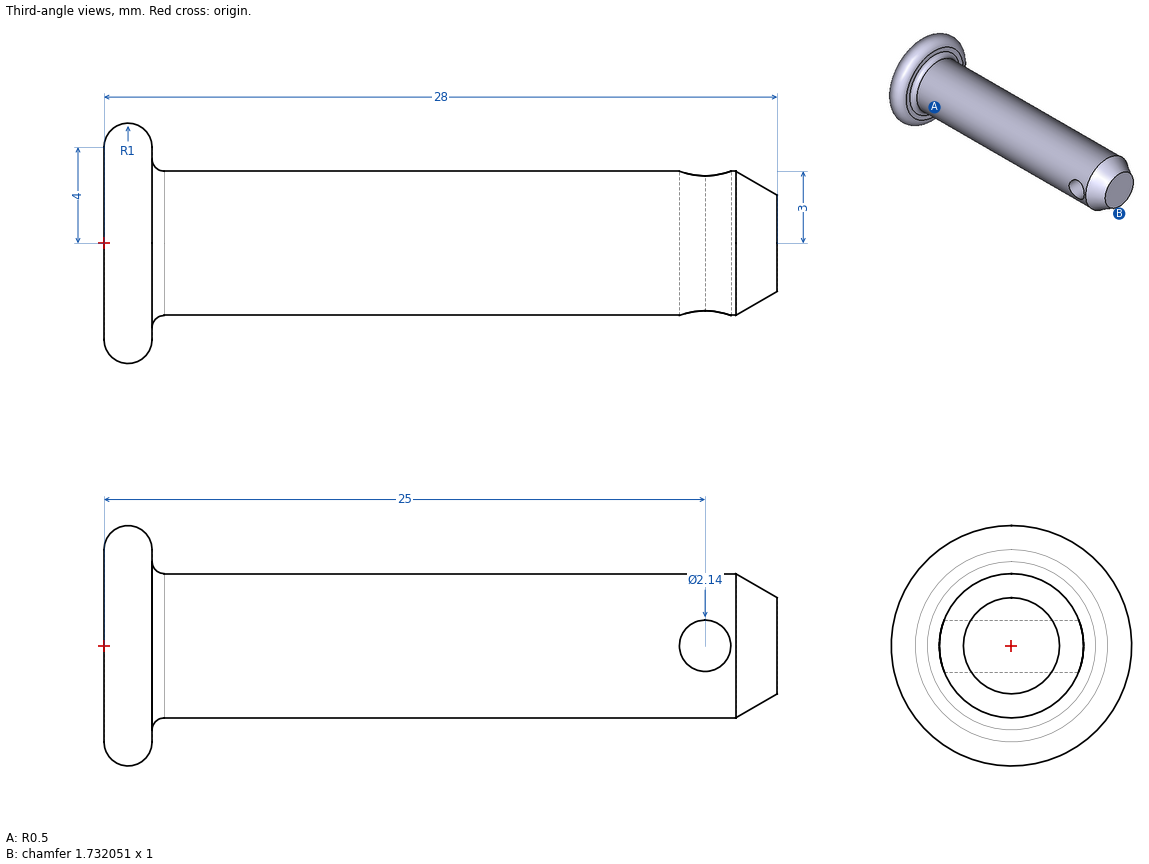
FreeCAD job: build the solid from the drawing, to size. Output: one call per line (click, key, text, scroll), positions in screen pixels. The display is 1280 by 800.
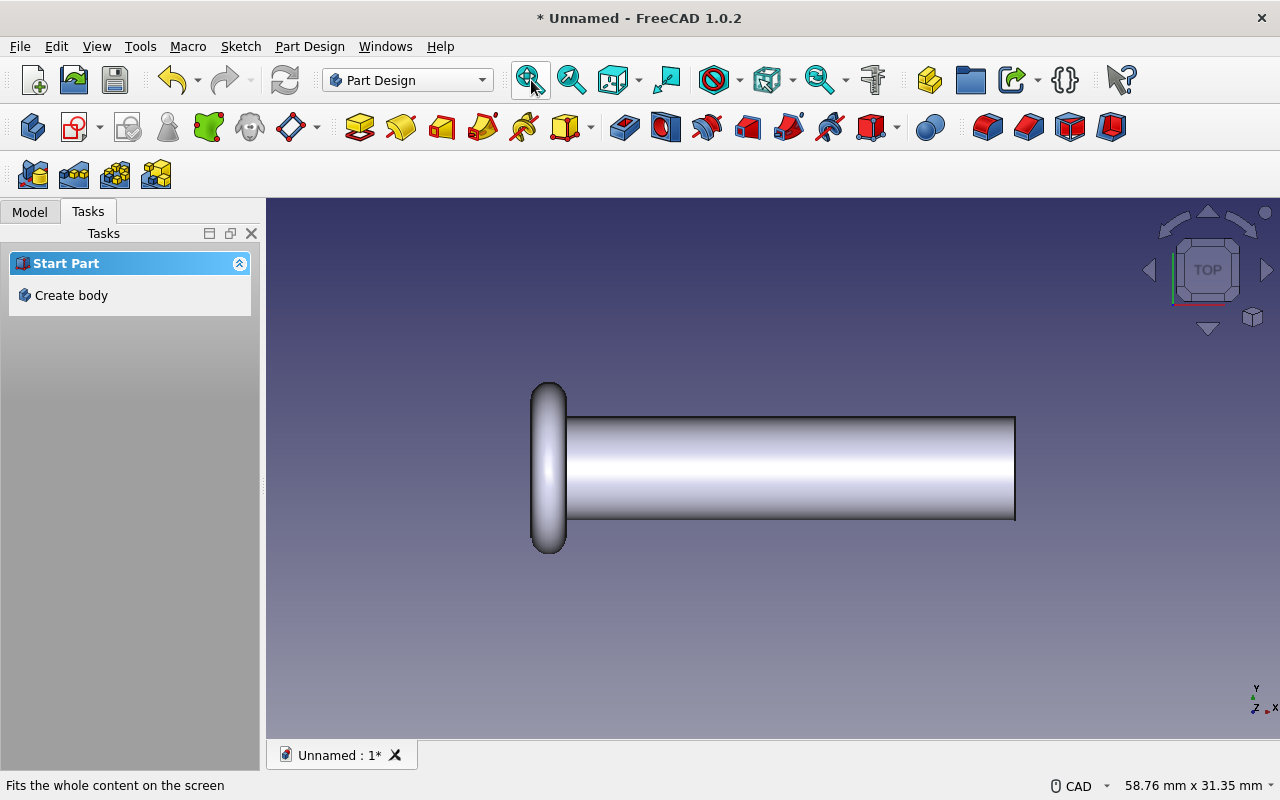
key(1)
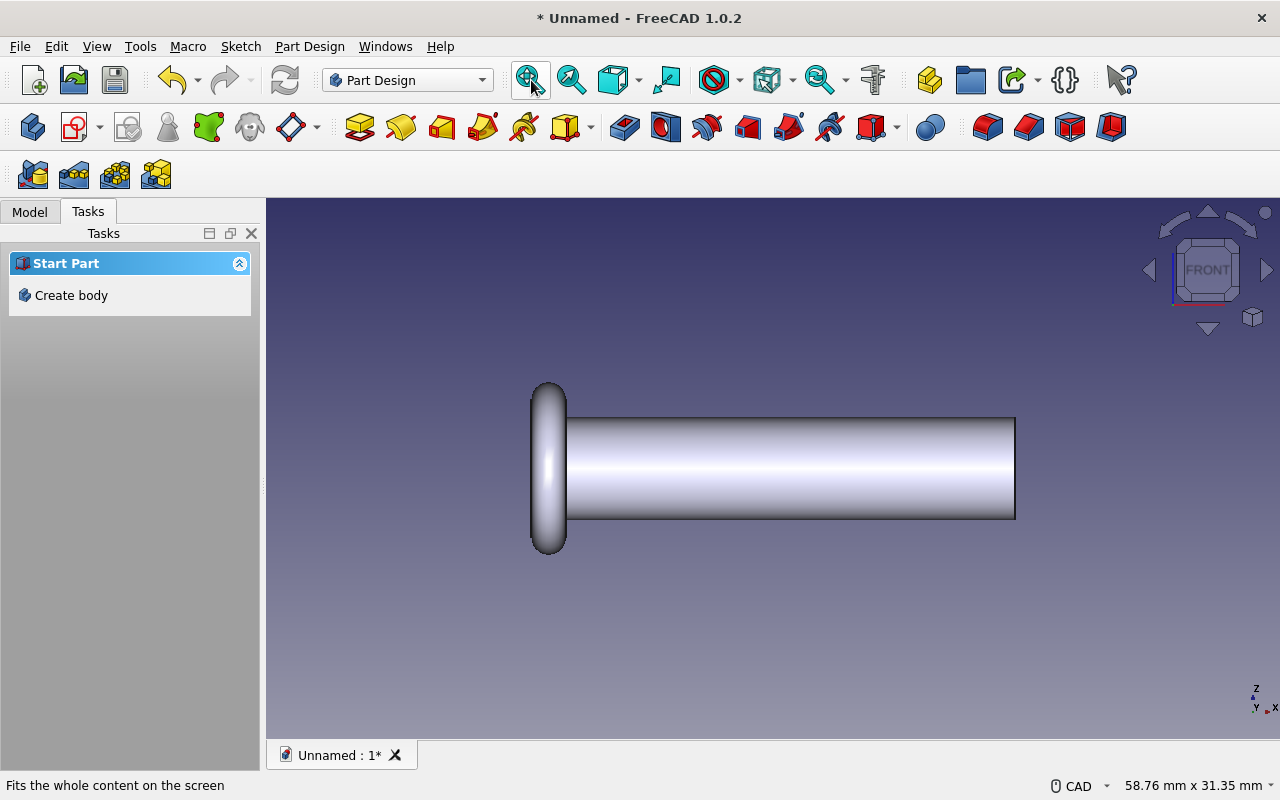
key(3)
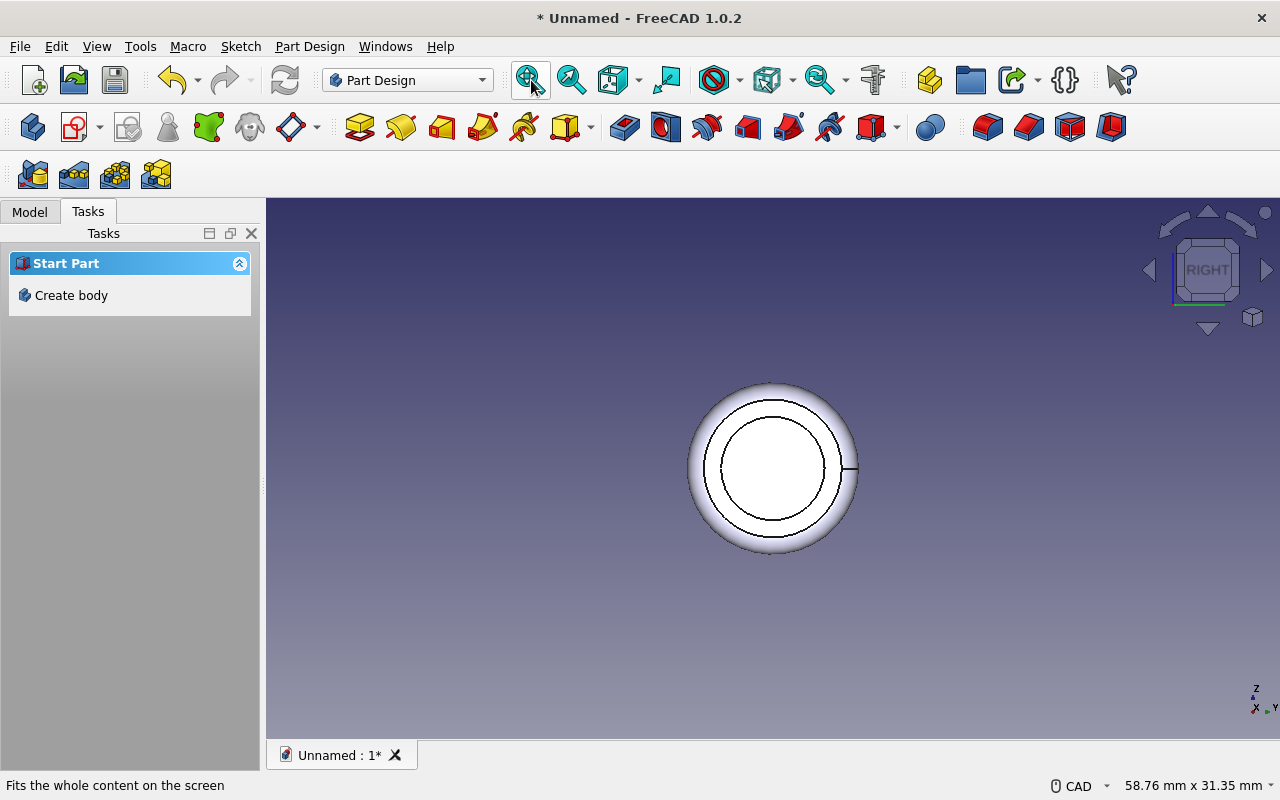
click(531, 80)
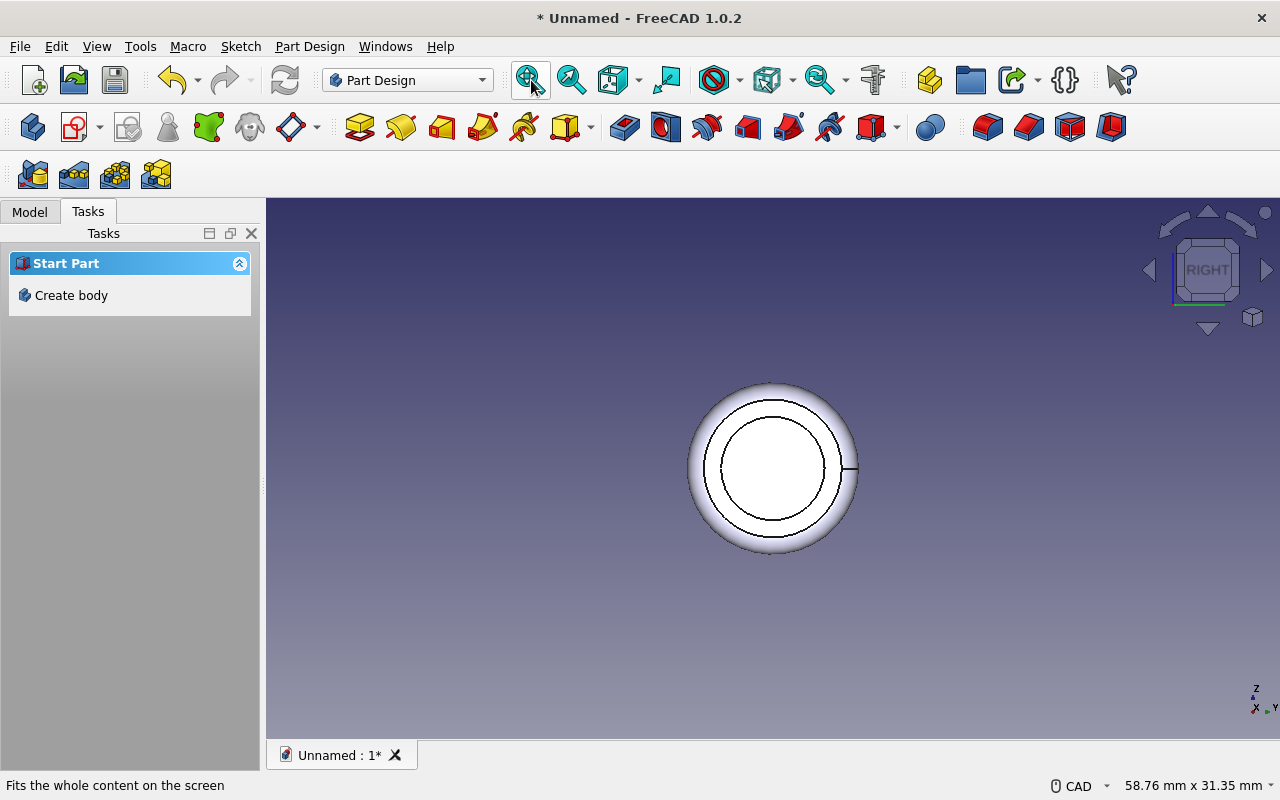
key(5)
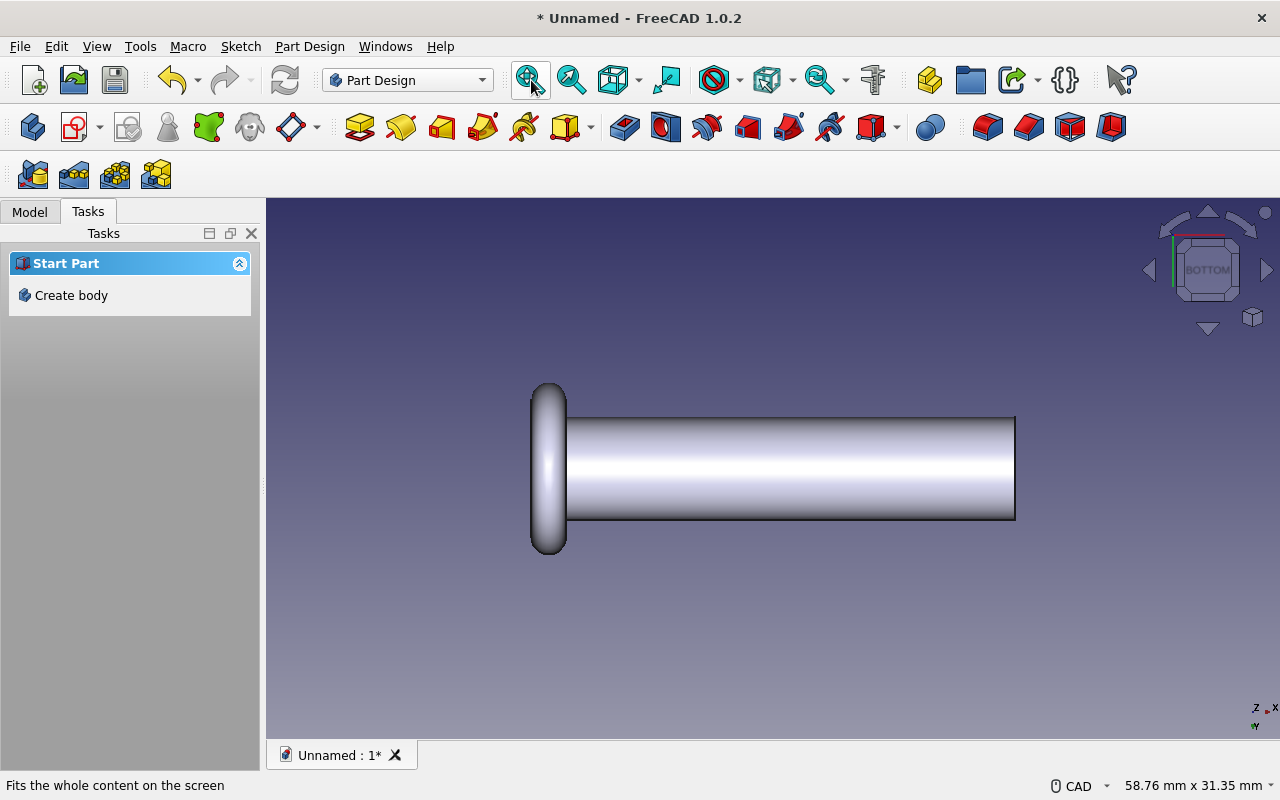
key(4)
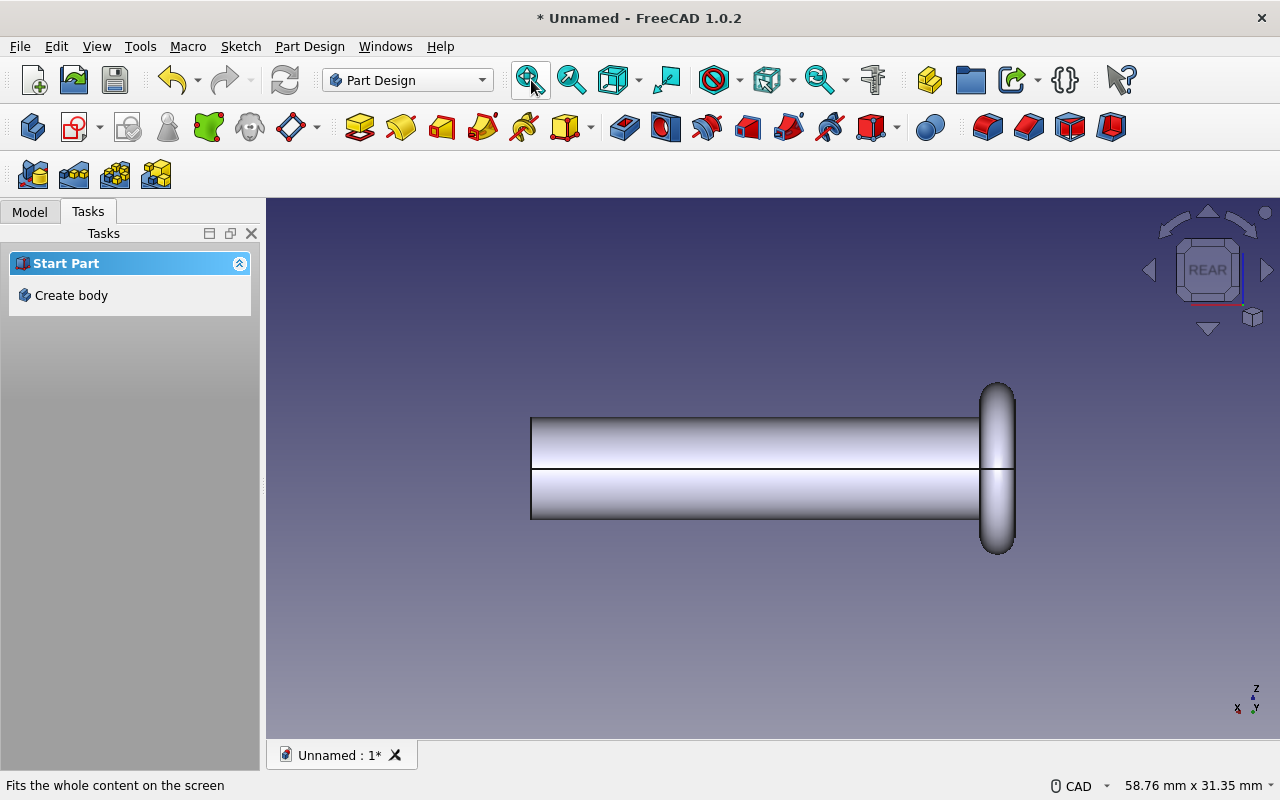
key(6)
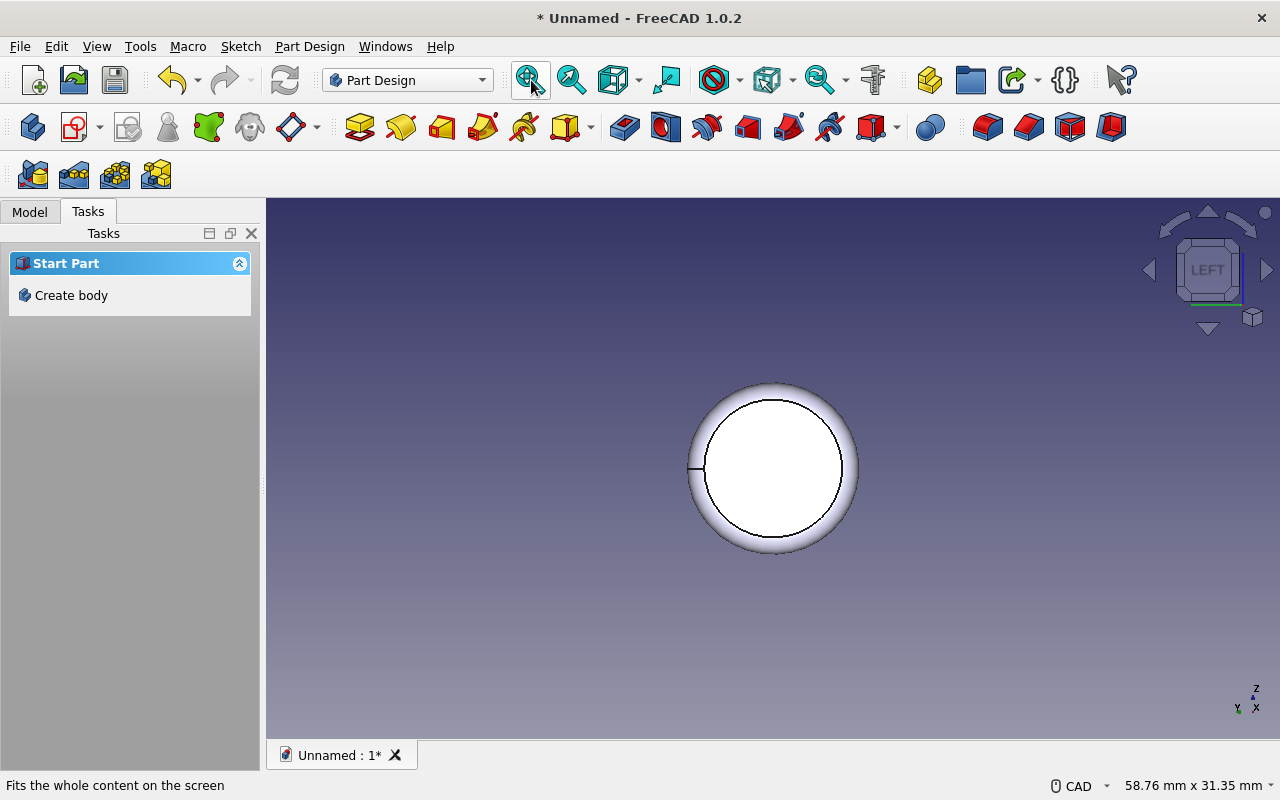
key(v)
key(f)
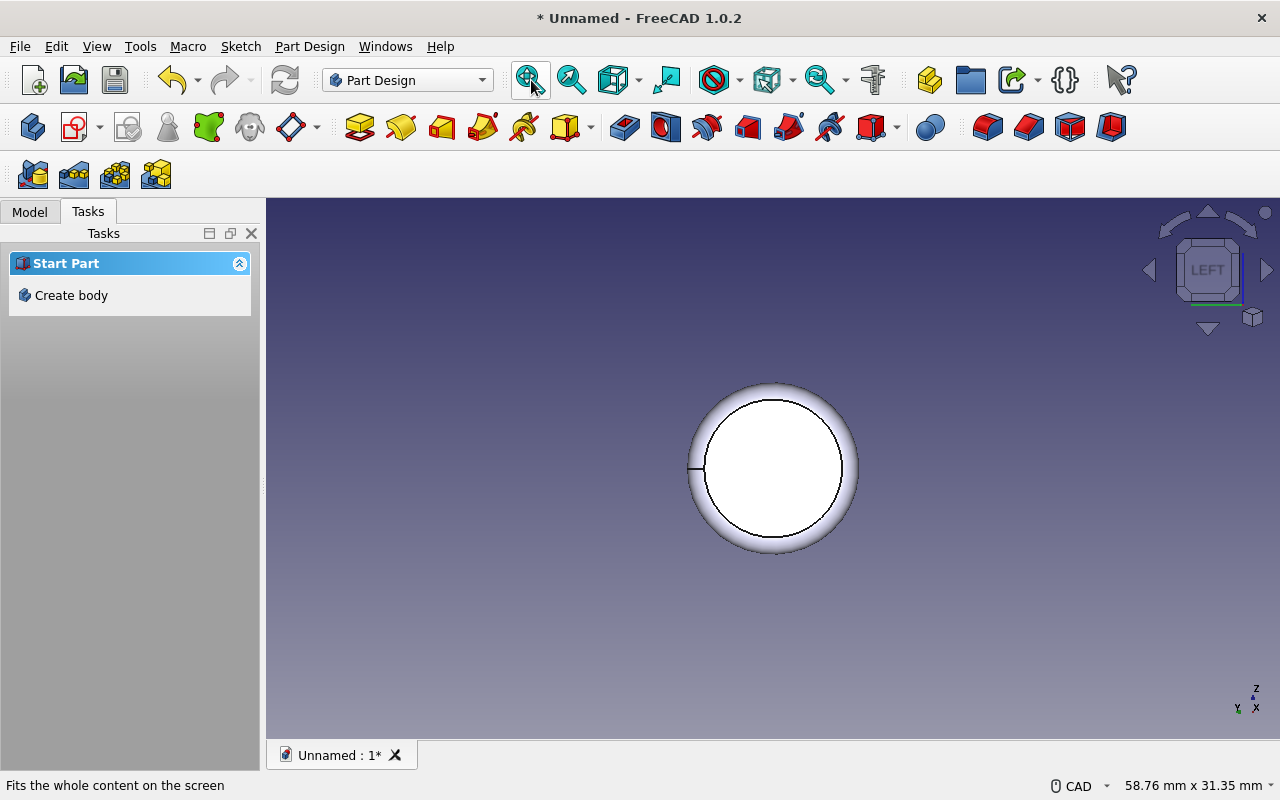
key(v)
key(3)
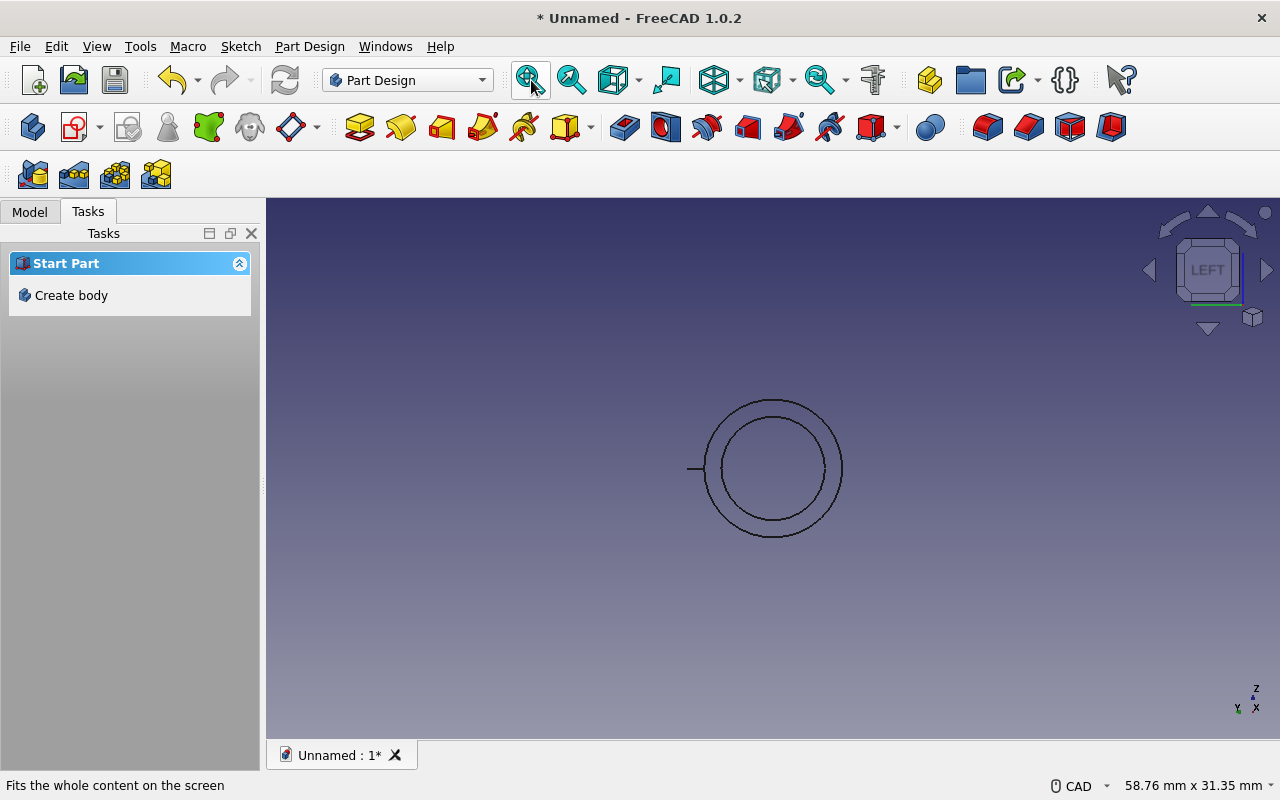
key(0)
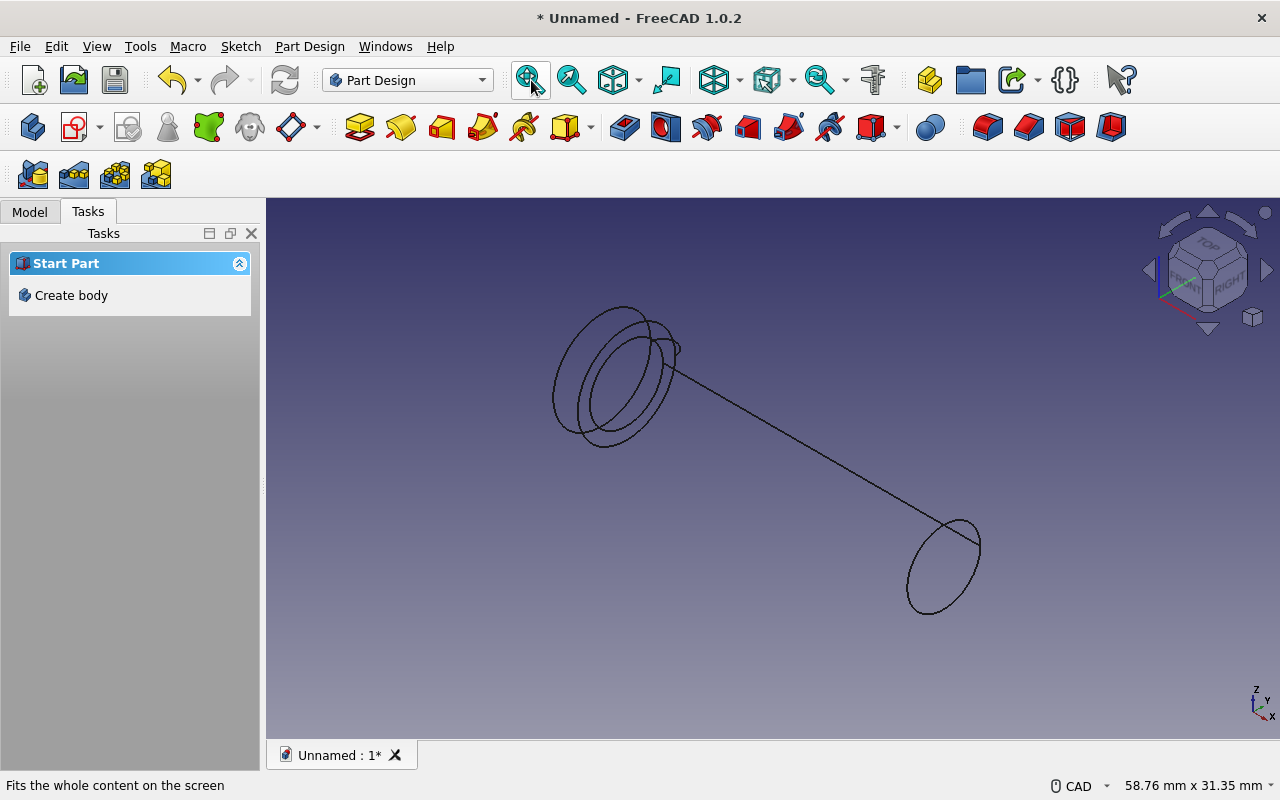
click(590, 404)